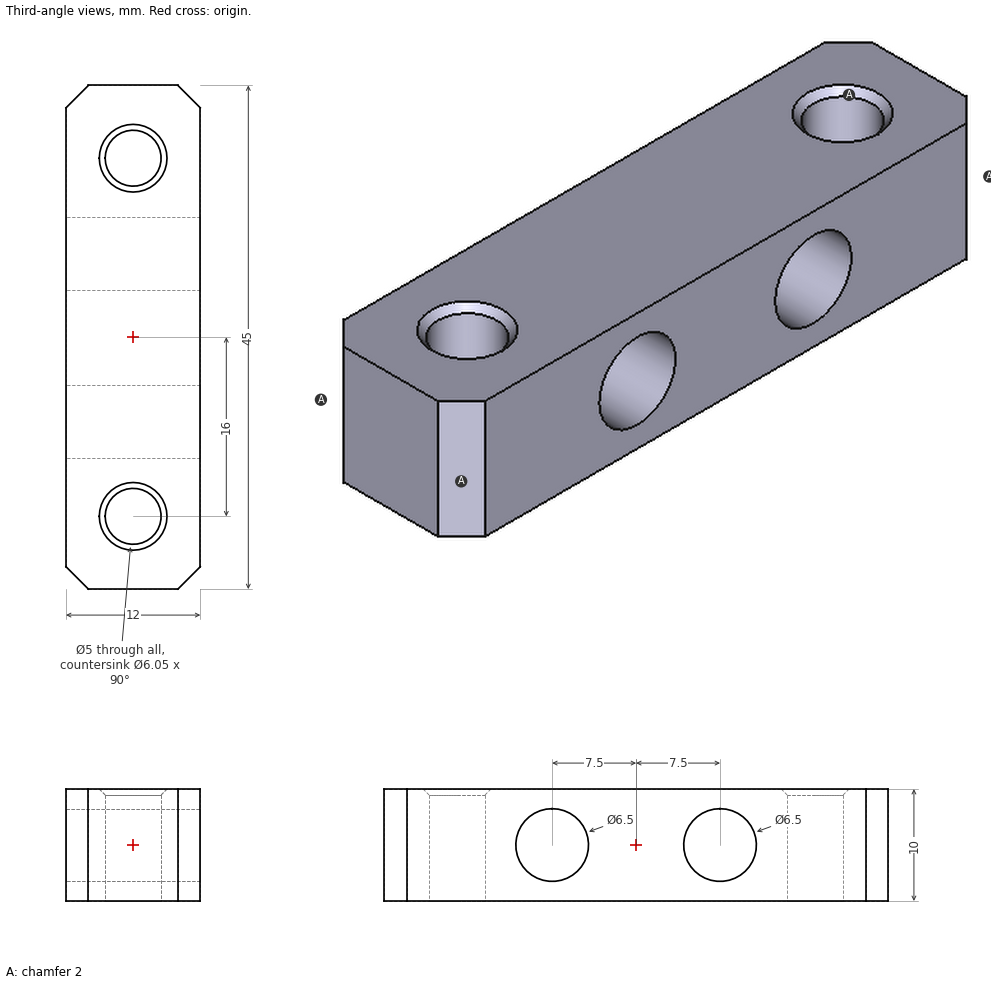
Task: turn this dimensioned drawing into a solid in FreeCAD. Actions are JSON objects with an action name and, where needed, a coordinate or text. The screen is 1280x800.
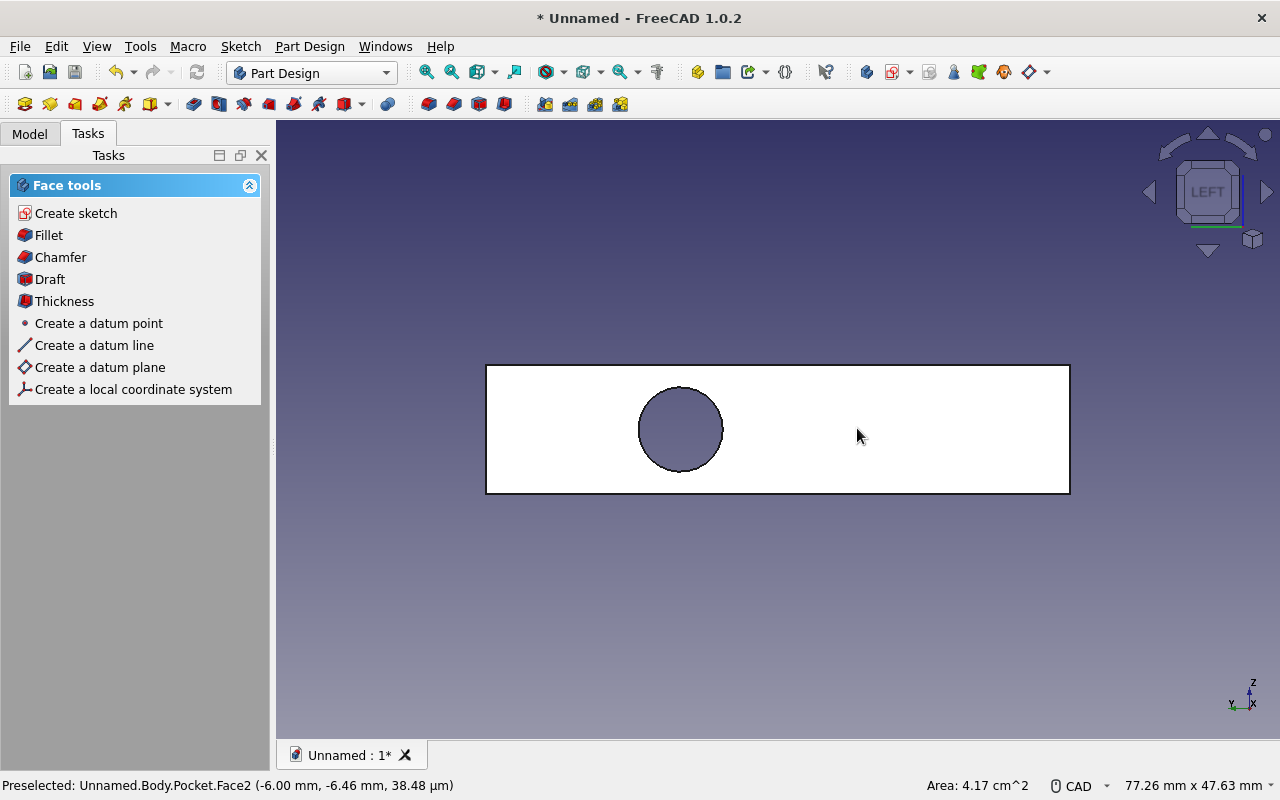
{"action": "left_click", "coordinate": [892, 72]}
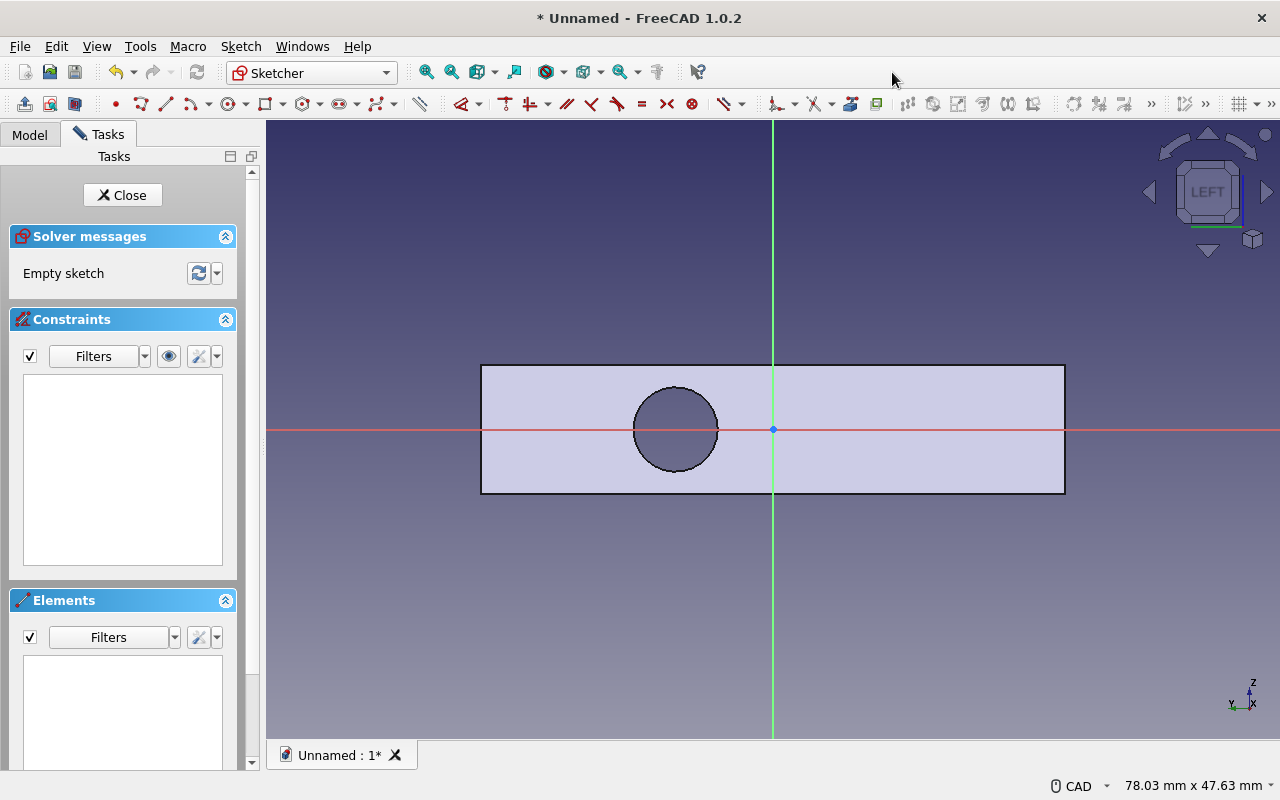
{"action": "scroll", "coordinate": [888, 430], "scroll_direction": "up", "scroll_amount": 7}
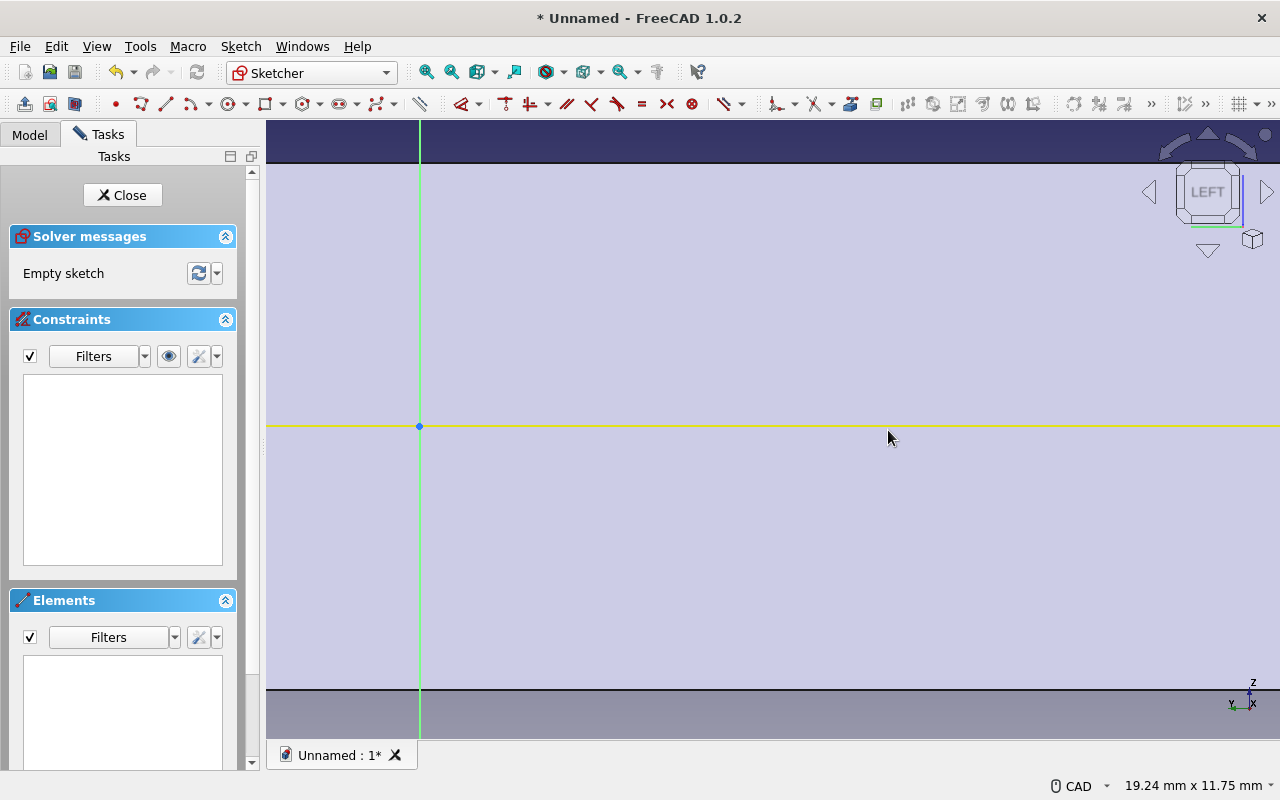
{"action": "left_click", "coordinate": [228, 104]}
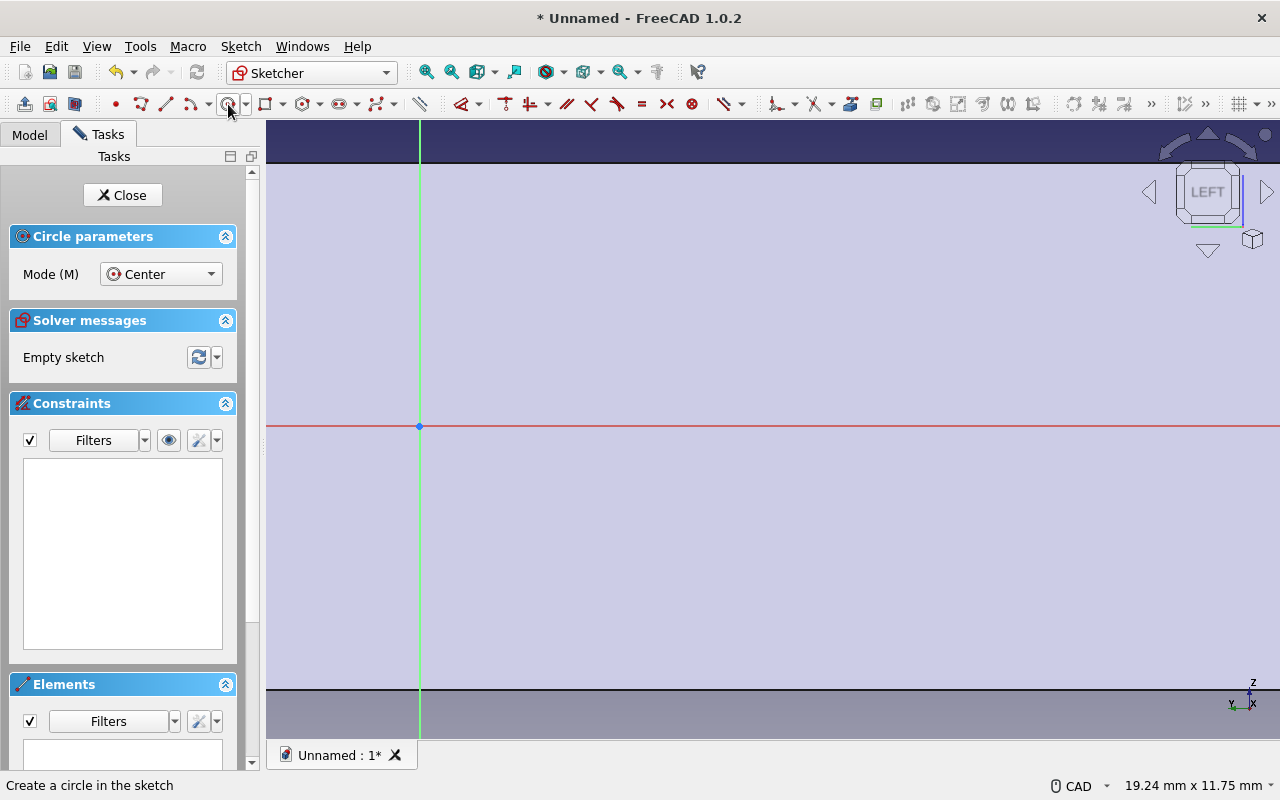
{"action": "left_click", "coordinate": [815, 426]}
{"action": "mouse_move", "coordinate": [936, 305]}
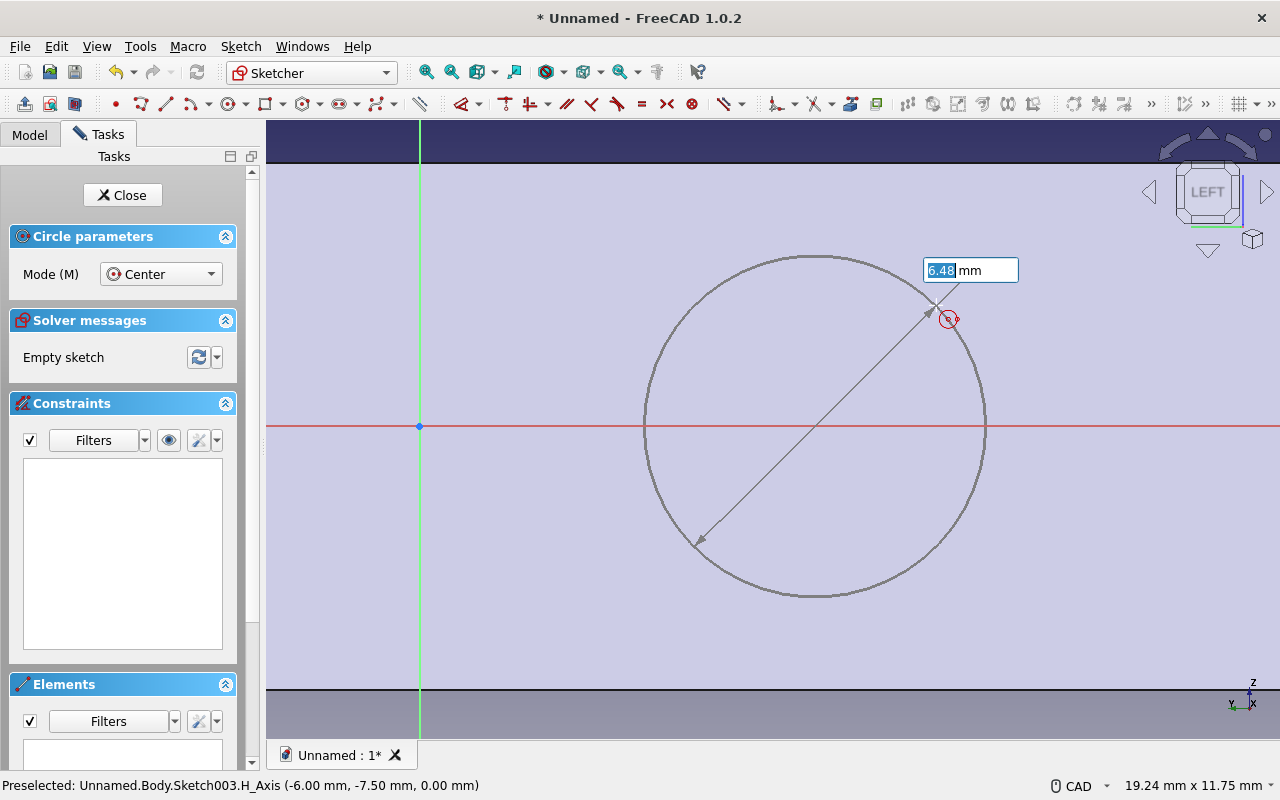
{"action": "type", "text": "6.5"}
{"action": "key", "text": "Return"}
{"action": "key", "text": "Escape"}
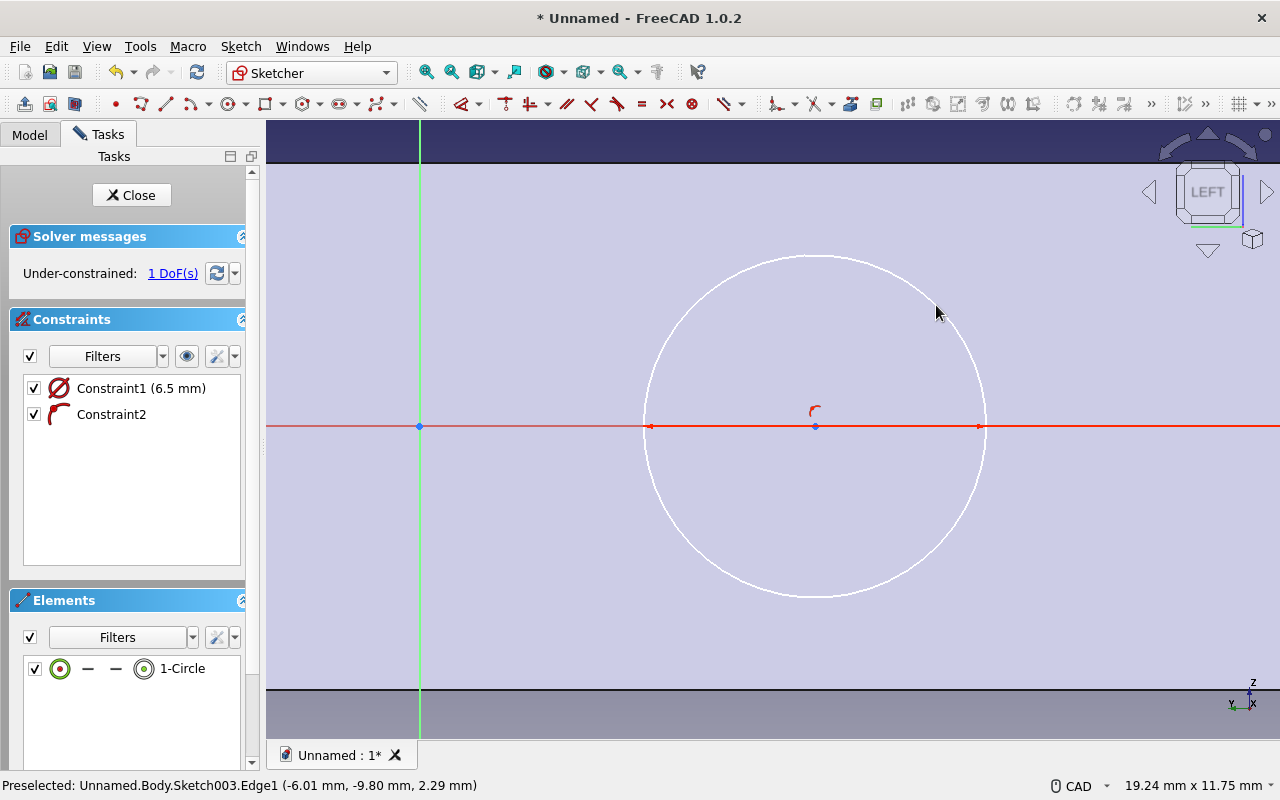
{"action": "left_click", "coordinate": [460, 104]}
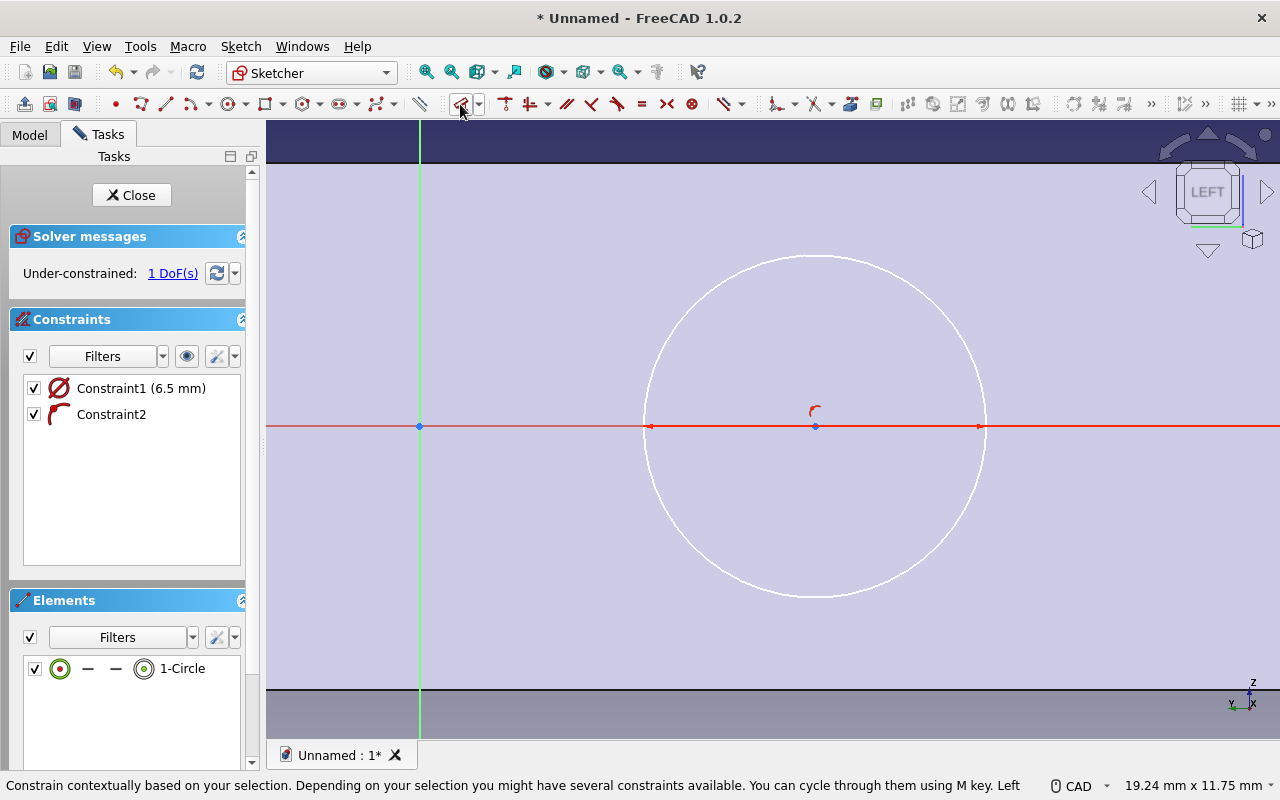
{"action": "left_click", "coordinate": [815, 426]}
{"action": "left_click", "coordinate": [617, 460]}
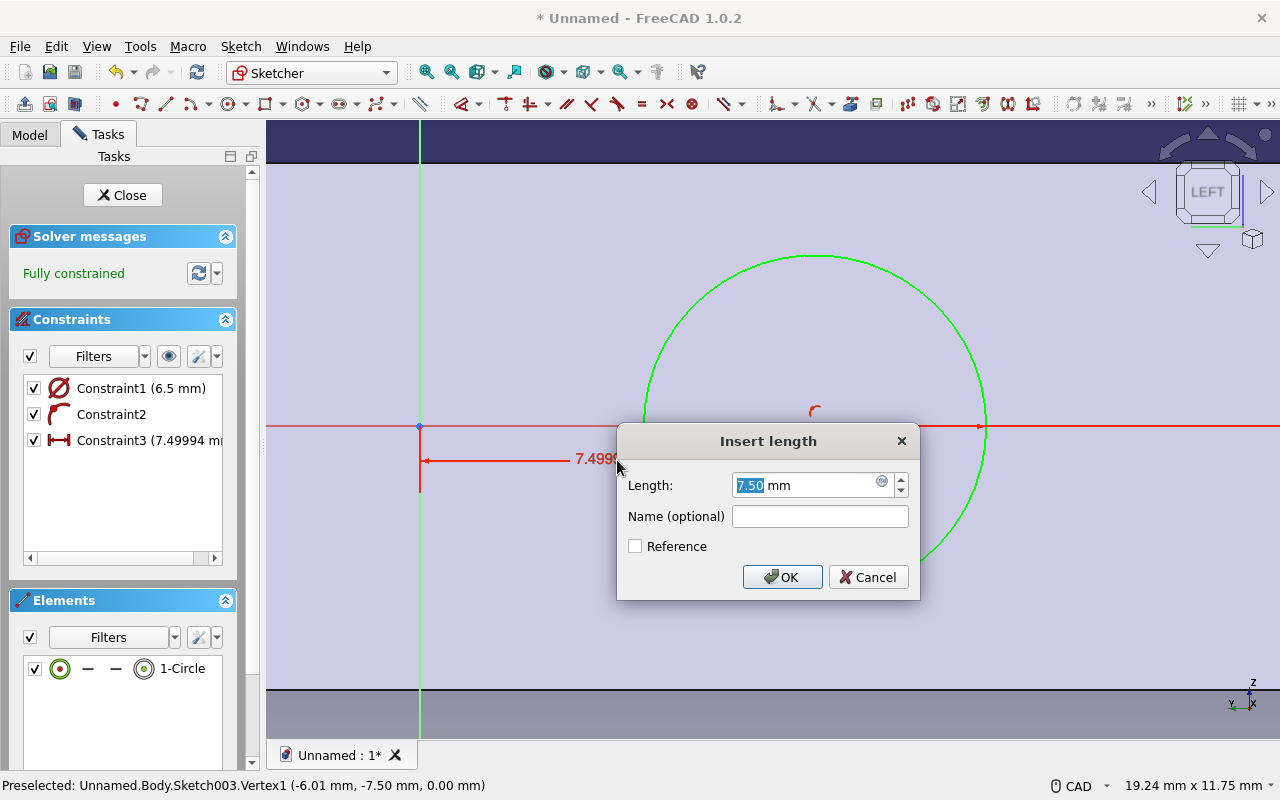
{"action": "type", "text": "7.5"}
{"action": "key", "text": "Return"}
{"action": "key", "text": "Escape"}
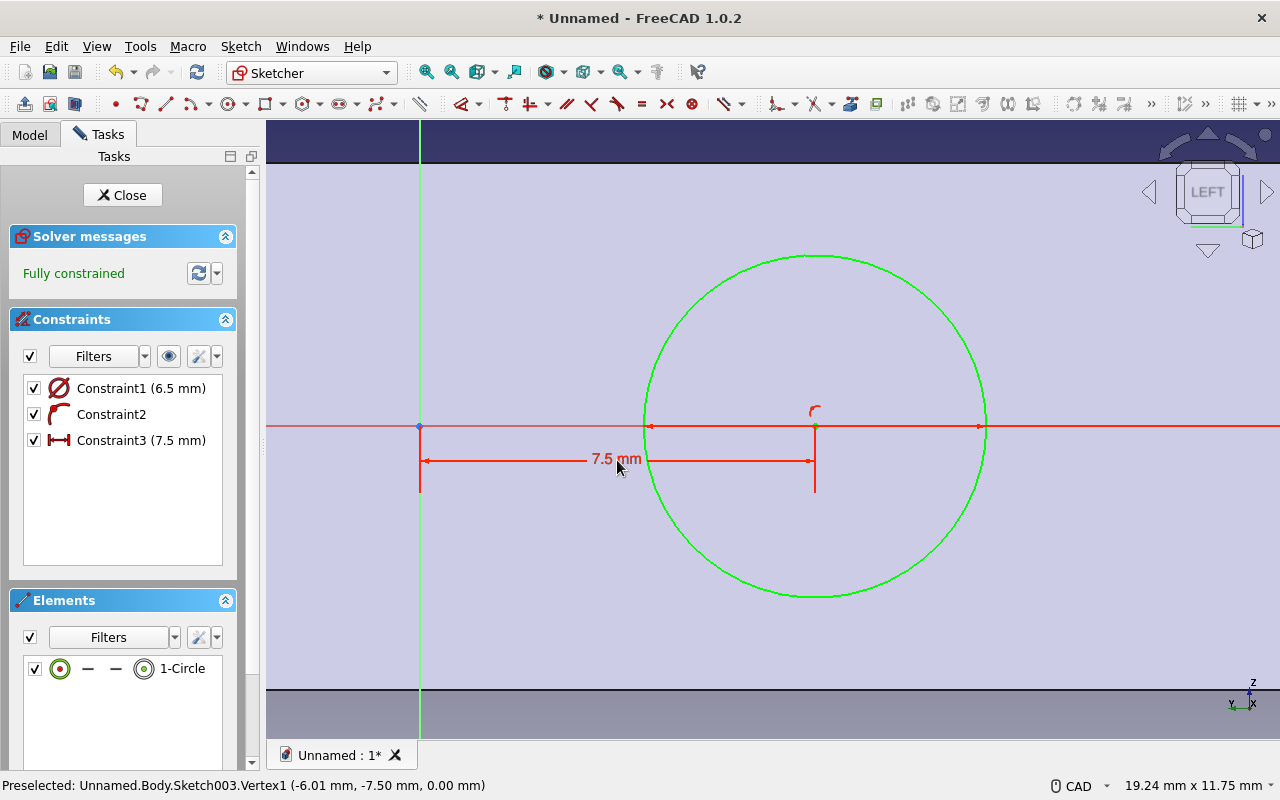
{"action": "left_click", "coordinate": [123, 195]}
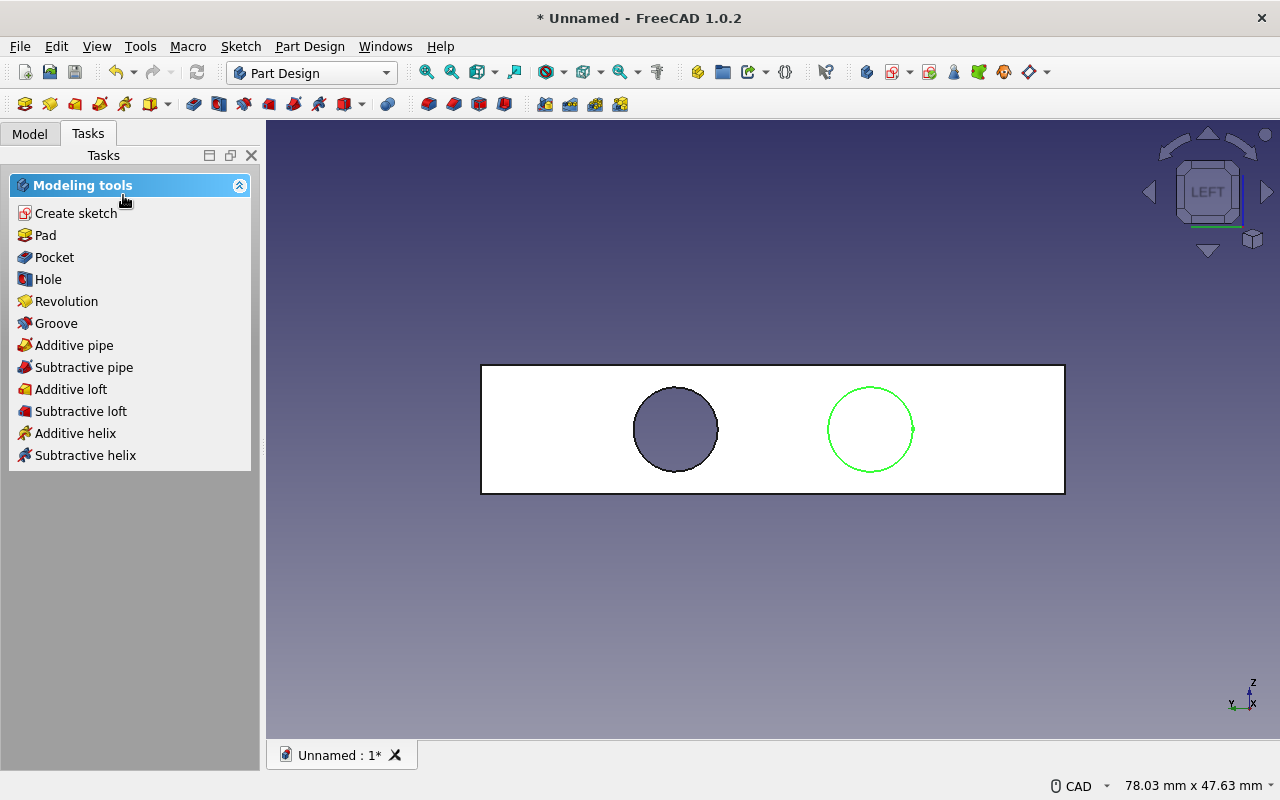
{"action": "left_click", "coordinate": [194, 104]}